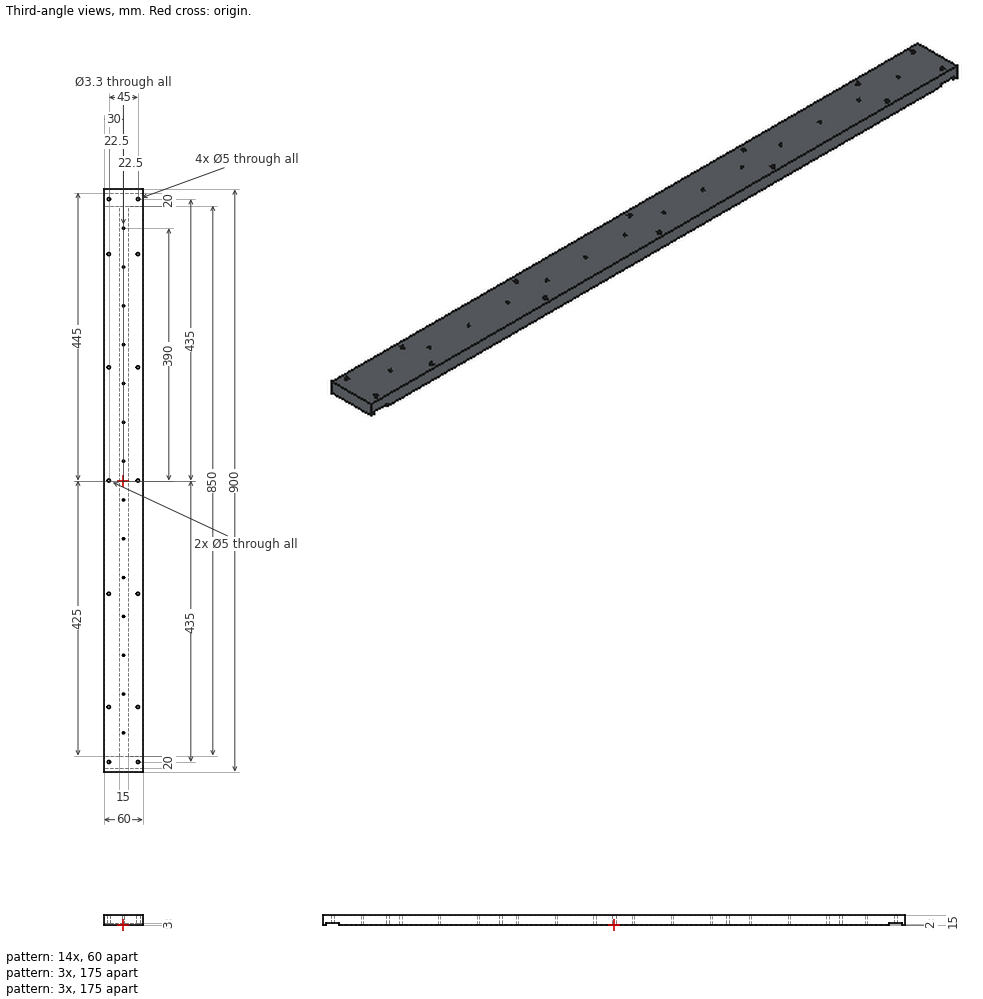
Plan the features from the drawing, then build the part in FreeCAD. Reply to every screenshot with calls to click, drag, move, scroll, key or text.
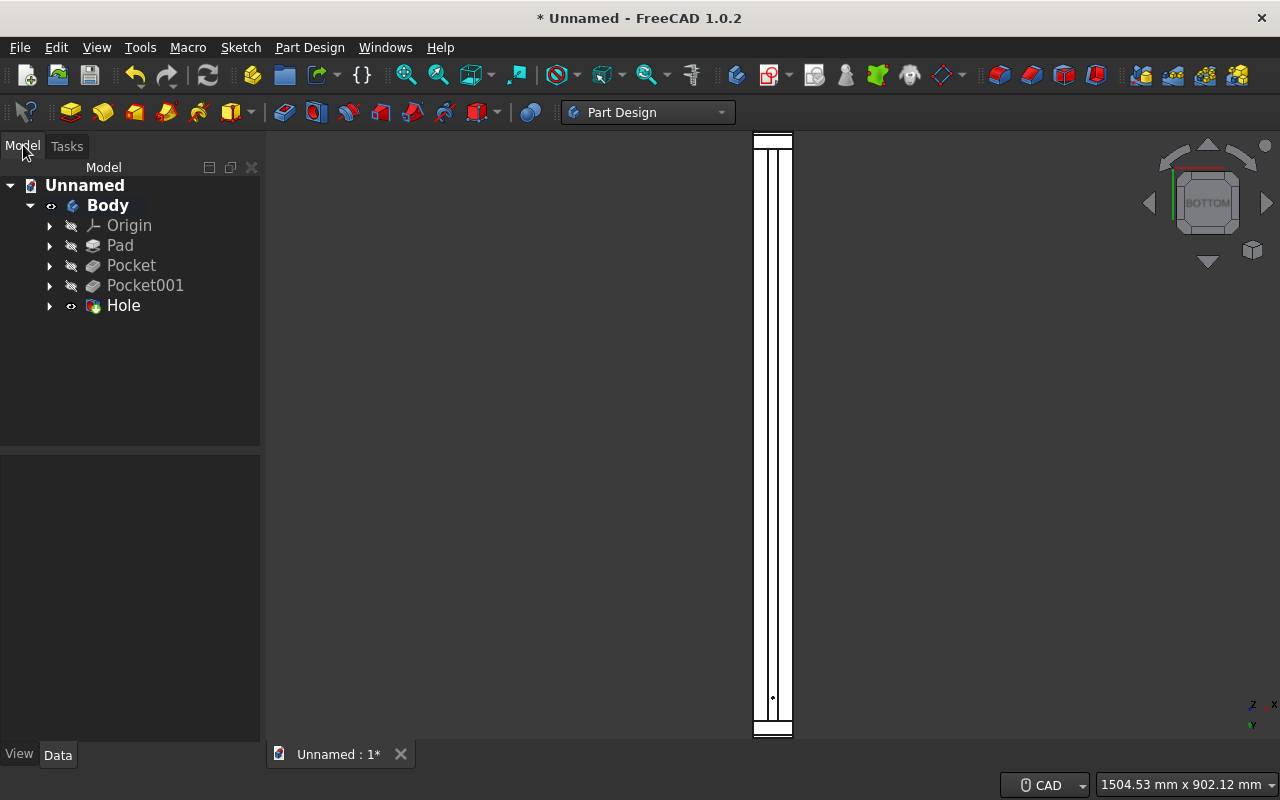
click(116, 306)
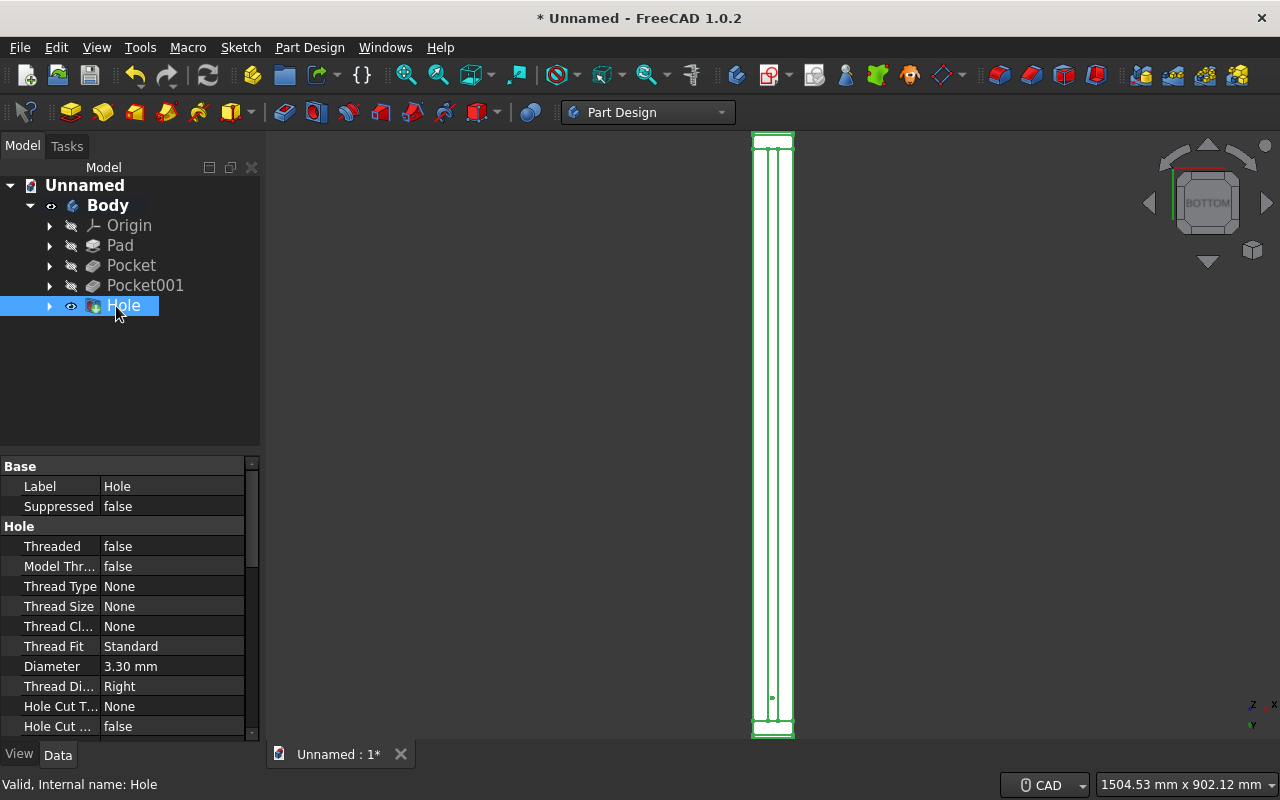
click(1174, 76)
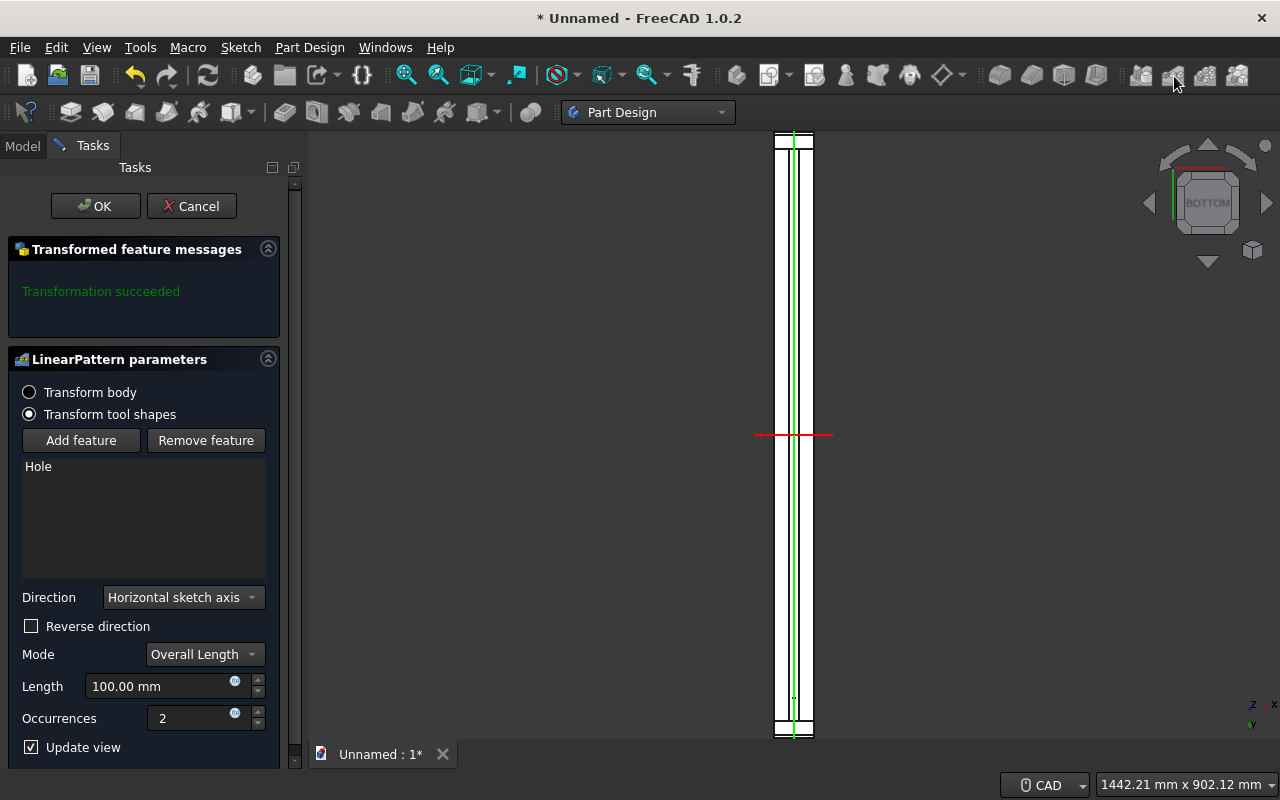
click(184, 598)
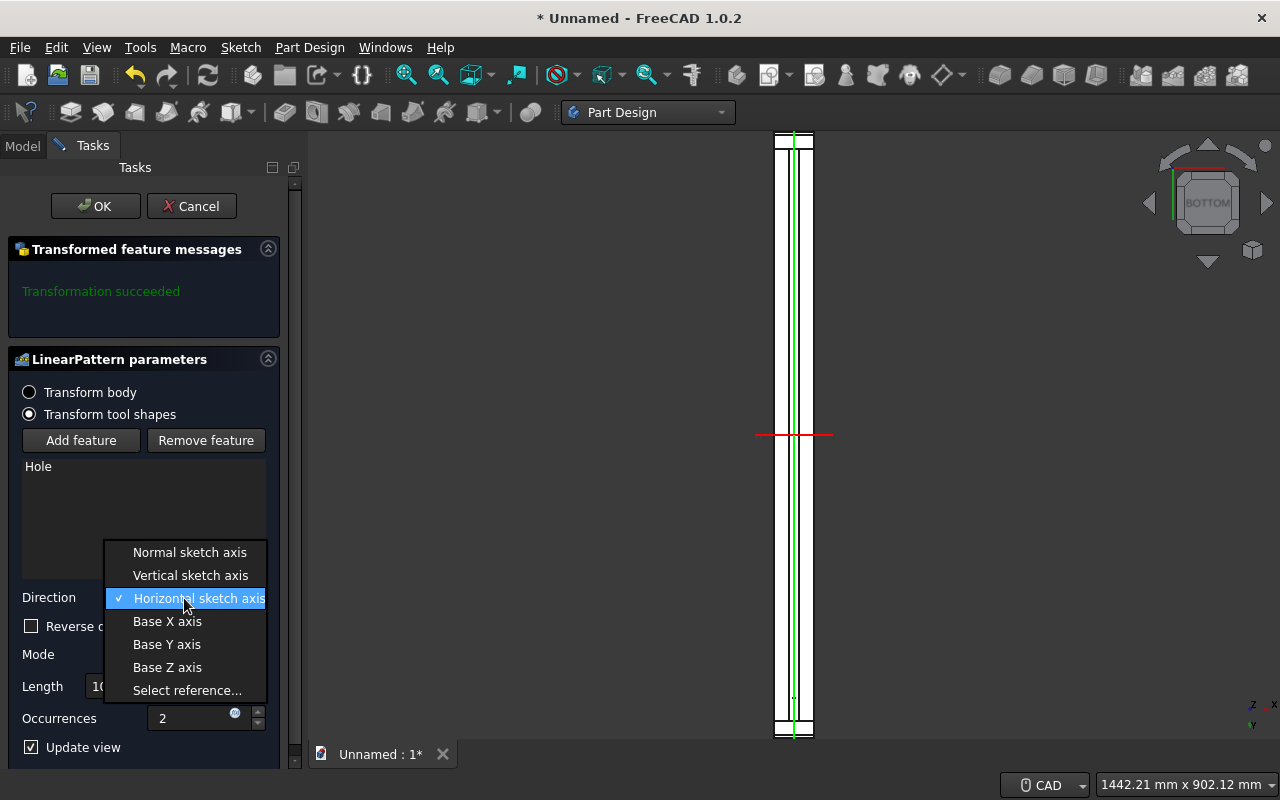
click(184, 644)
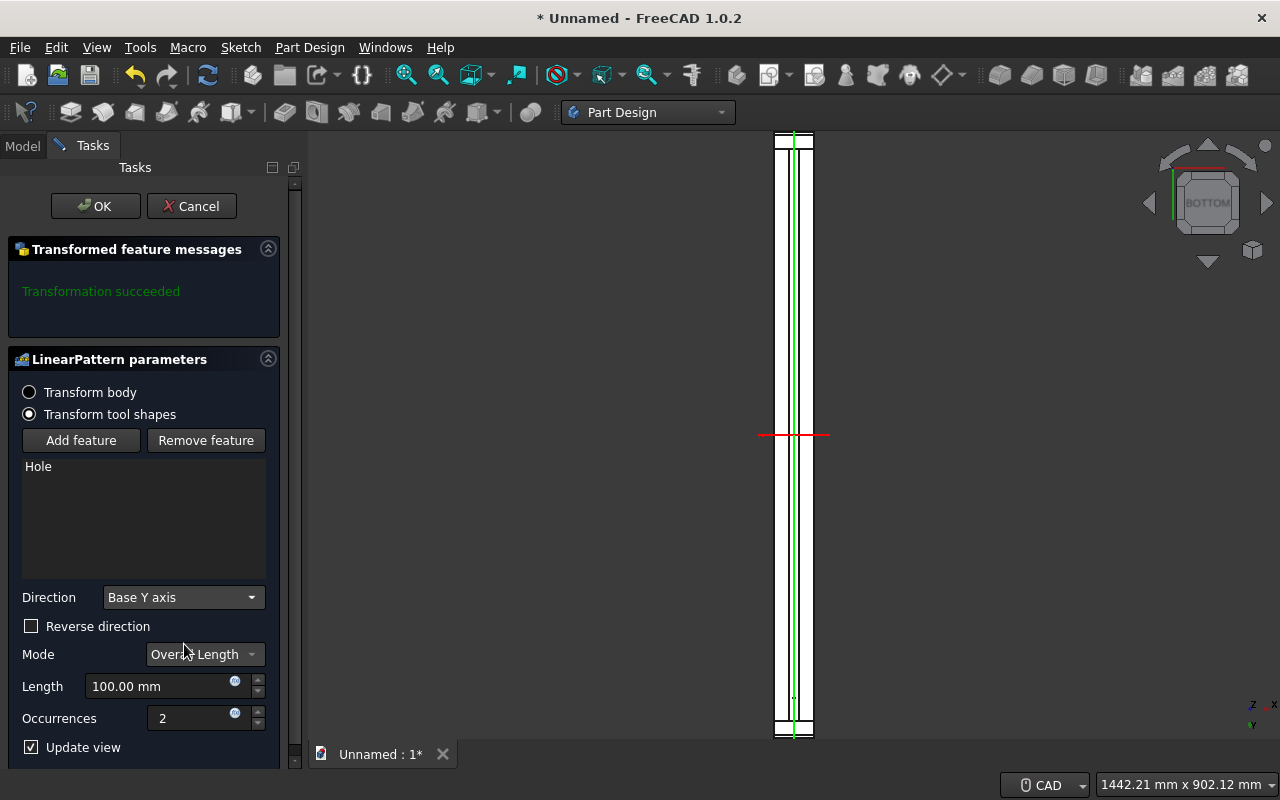
click(206, 654)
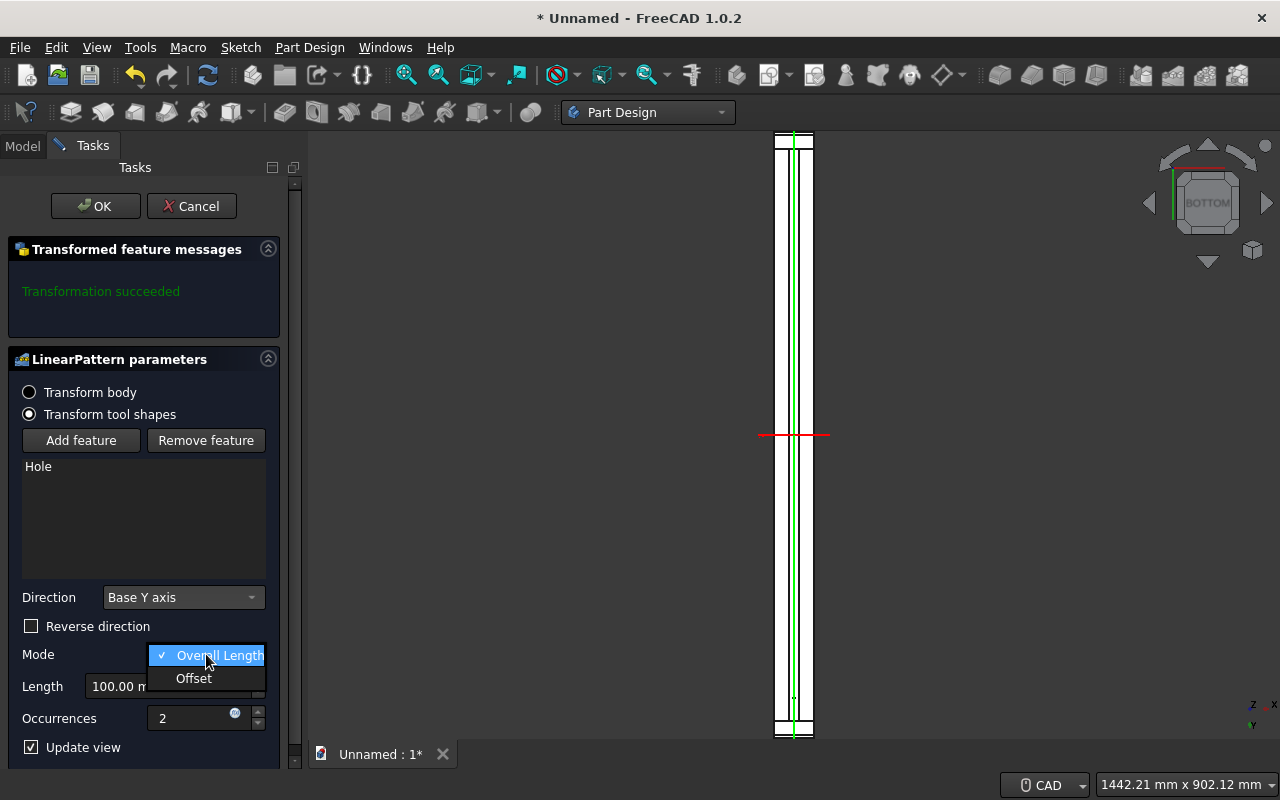
click(206, 678)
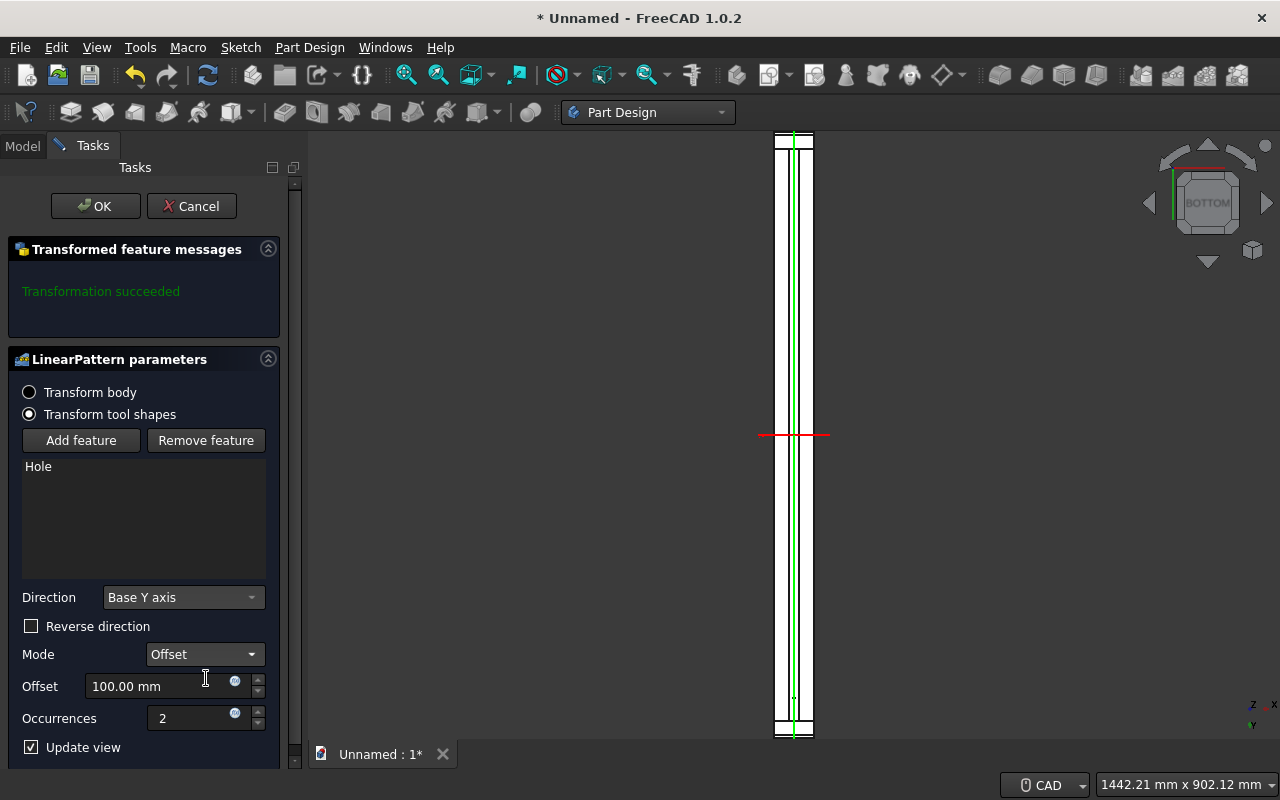
triple_click(168, 686)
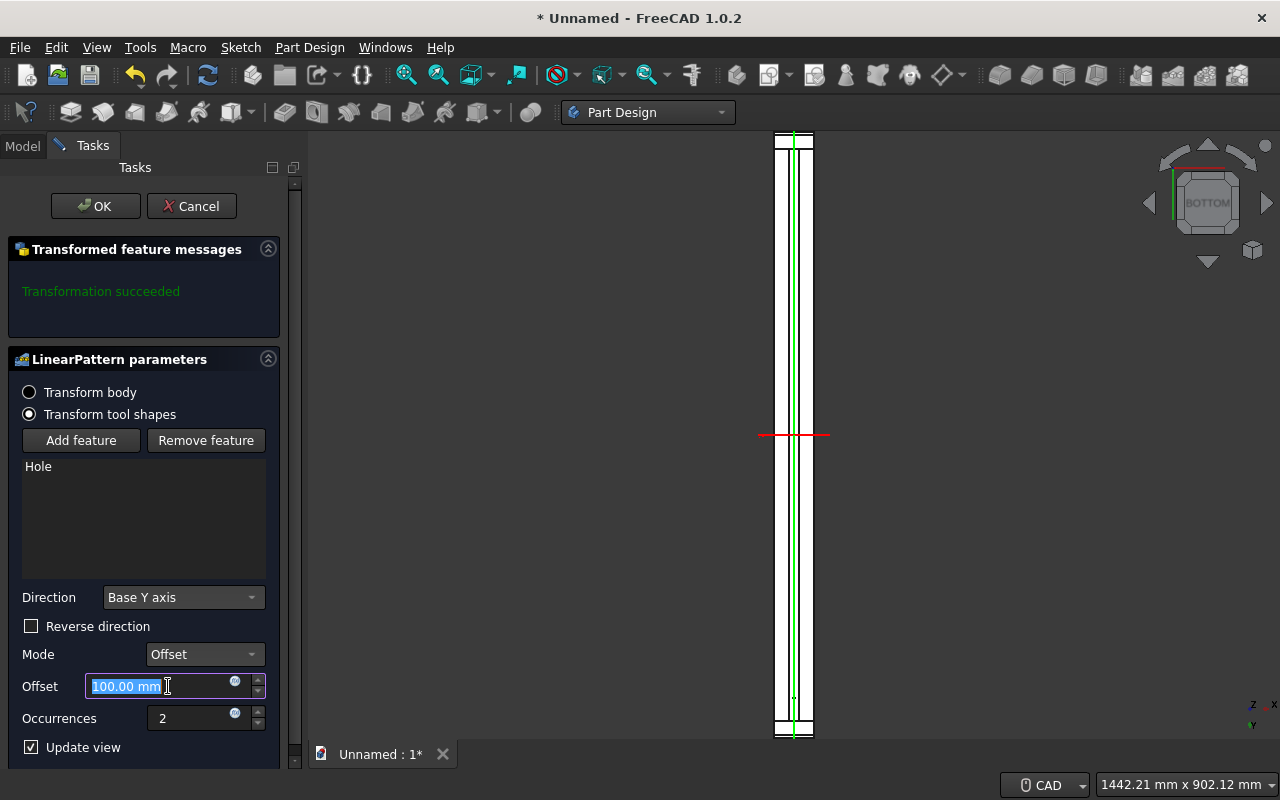
text(60)
key(Tab)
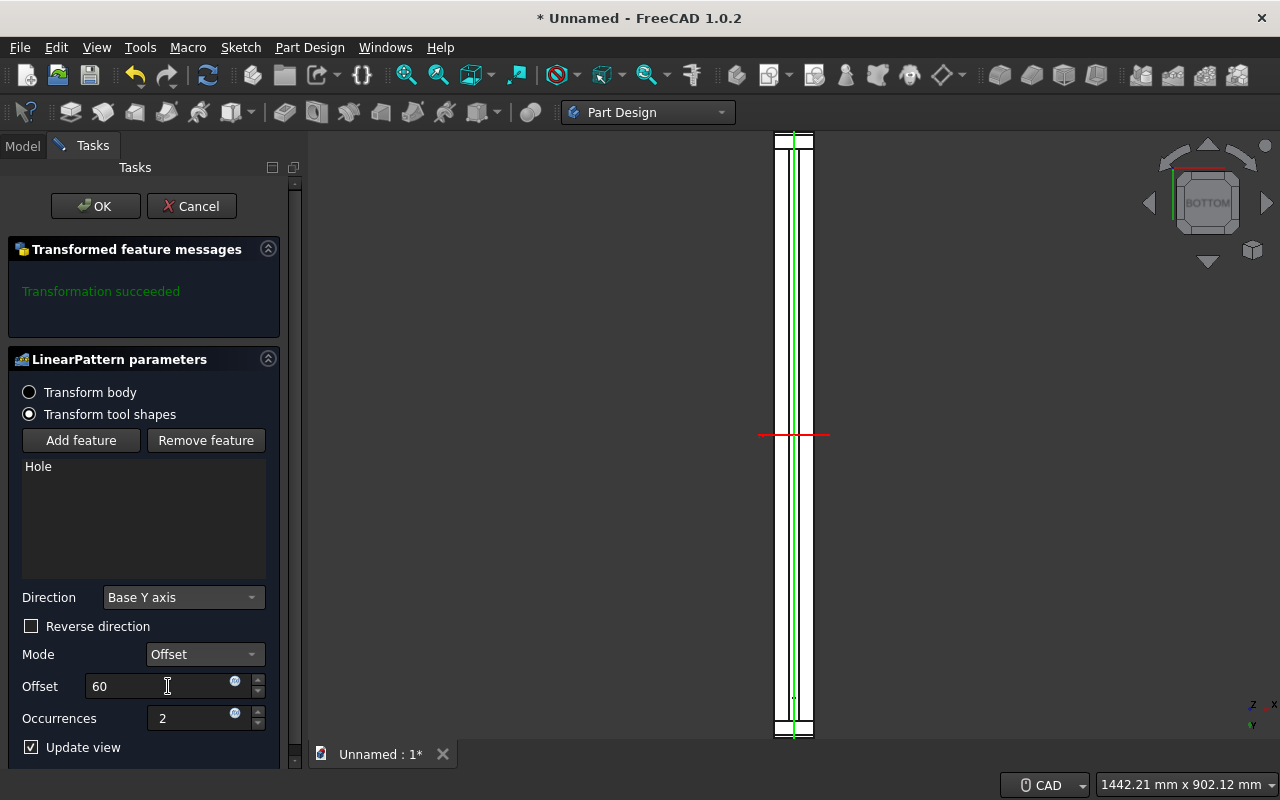
triple_click(198, 718)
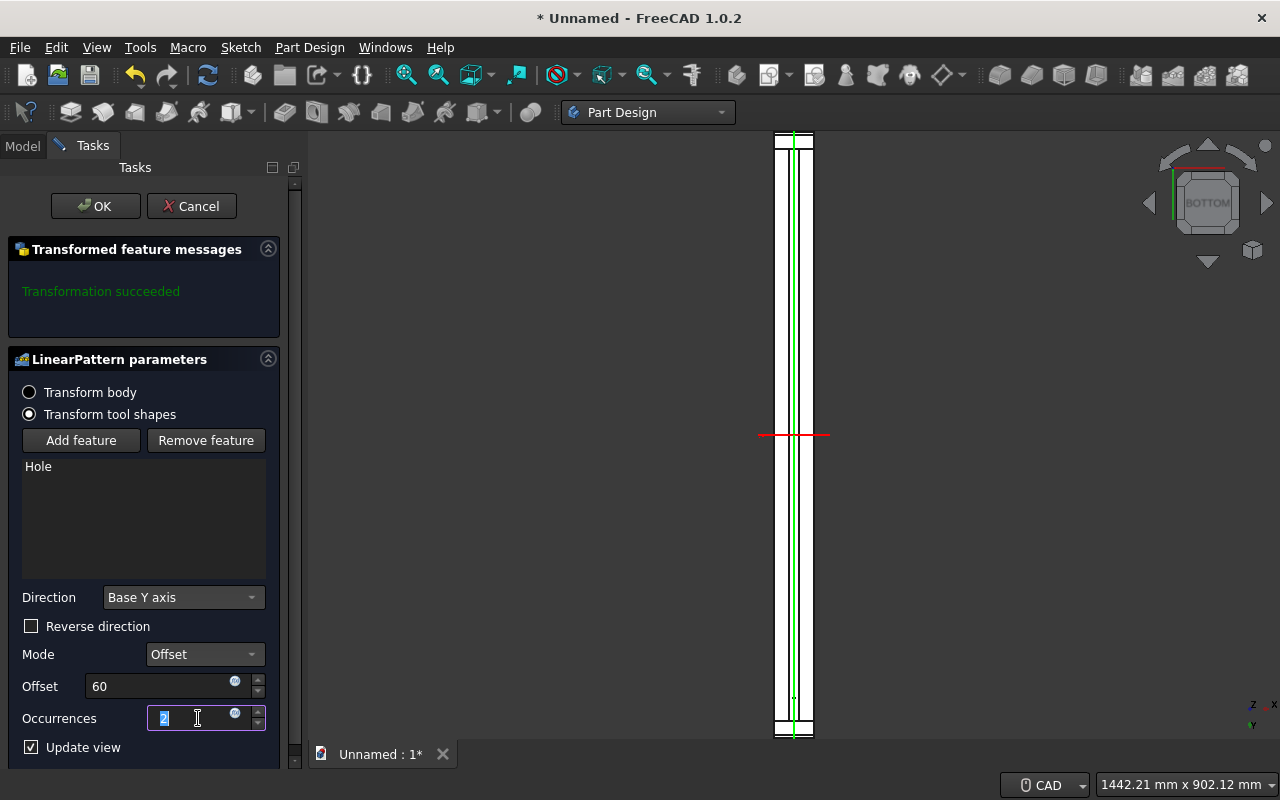
text(14)
key(Tab)